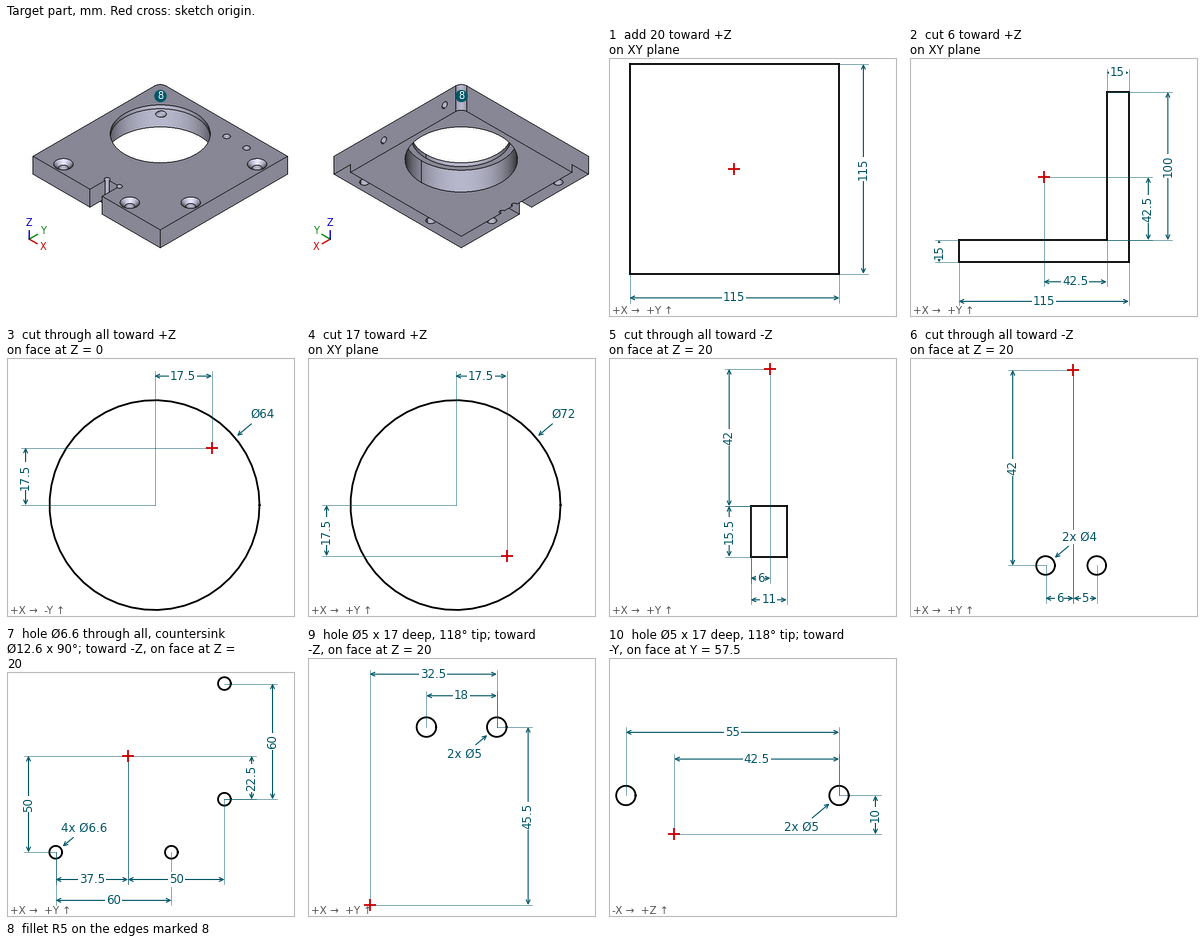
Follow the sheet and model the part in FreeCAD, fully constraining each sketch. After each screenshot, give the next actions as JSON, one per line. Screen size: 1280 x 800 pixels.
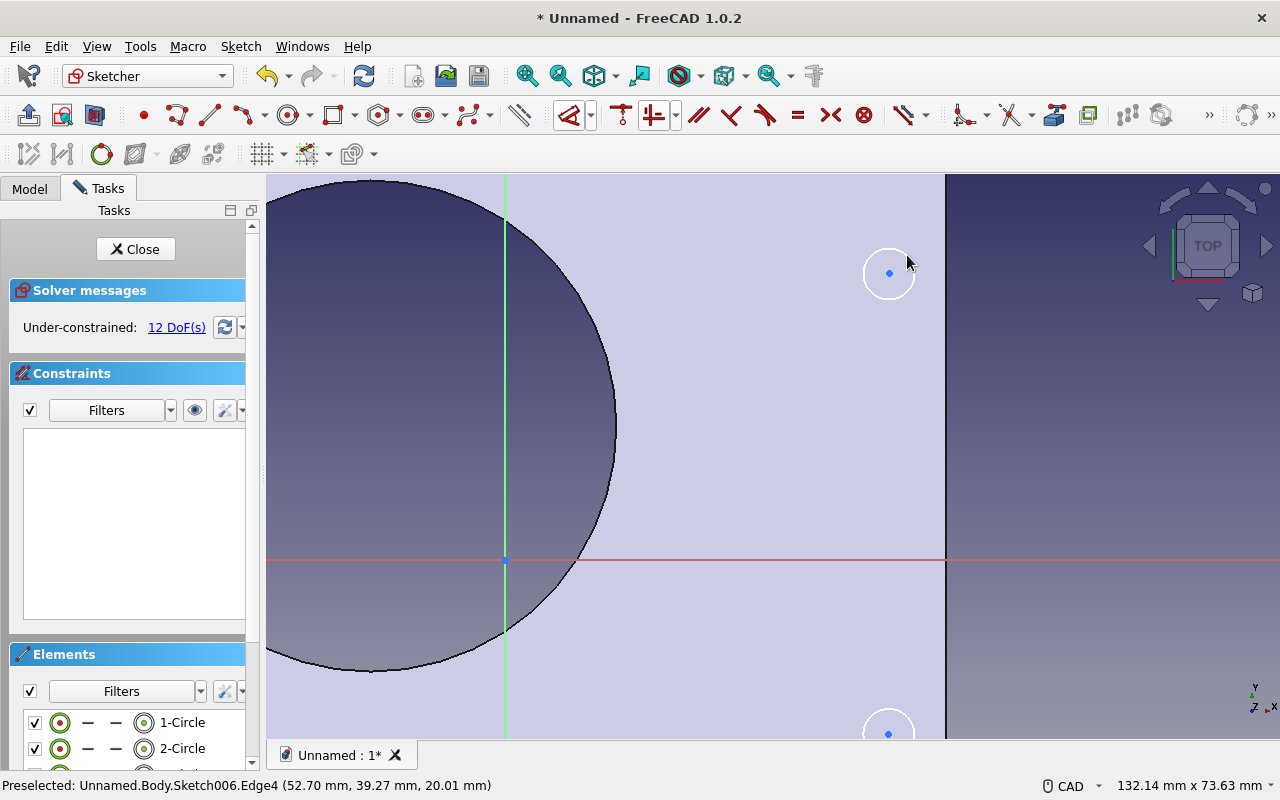
{"action": "scroll", "coordinate": [889, 272], "scroll_direction": "down", "scroll_amount": 3}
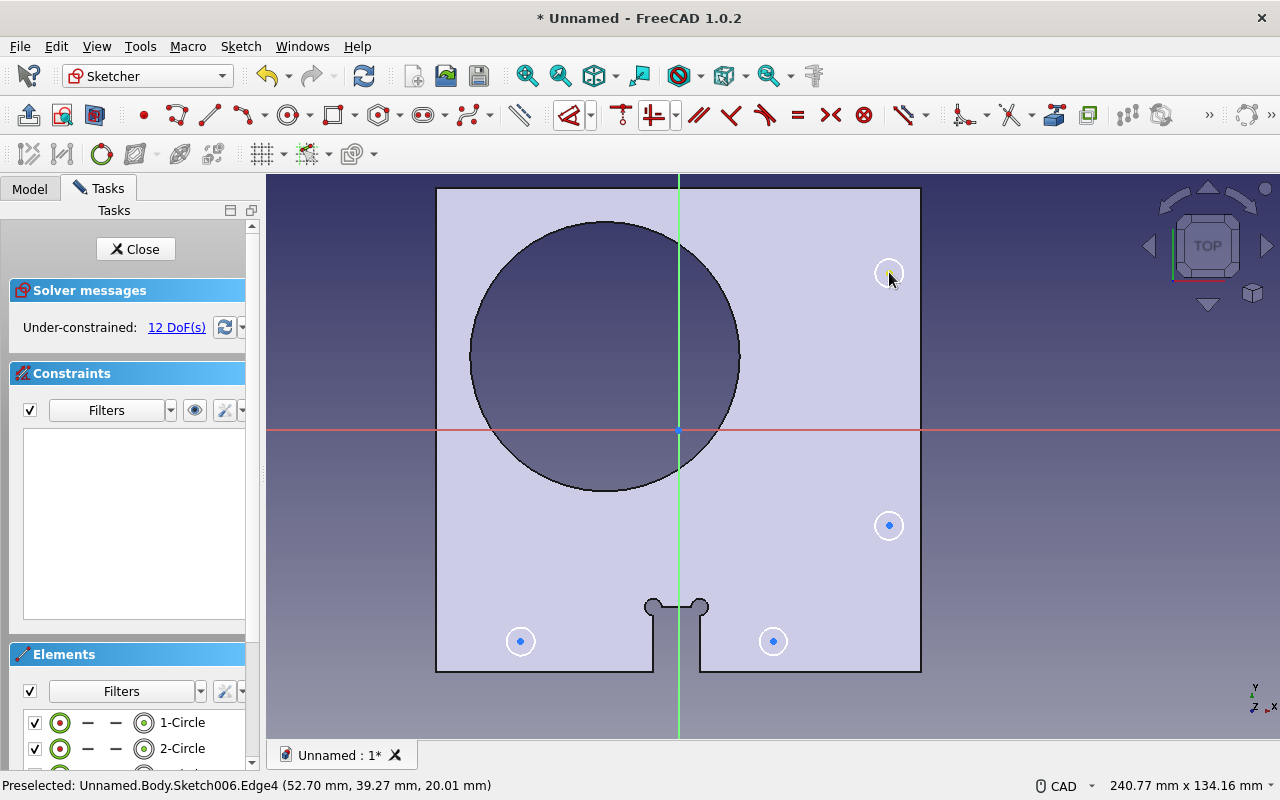
{"action": "left_click", "coordinate": [531, 632]}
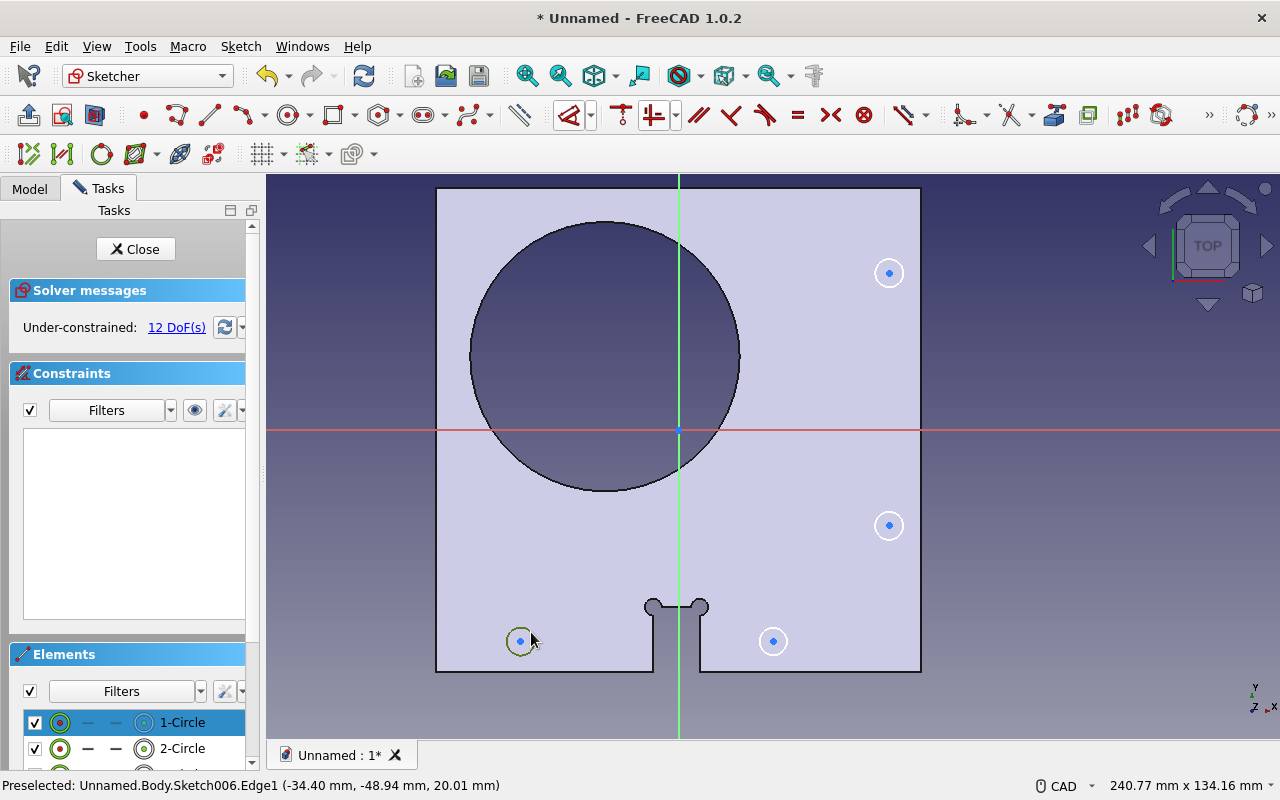
{"action": "left_click", "coordinate": [783, 632]}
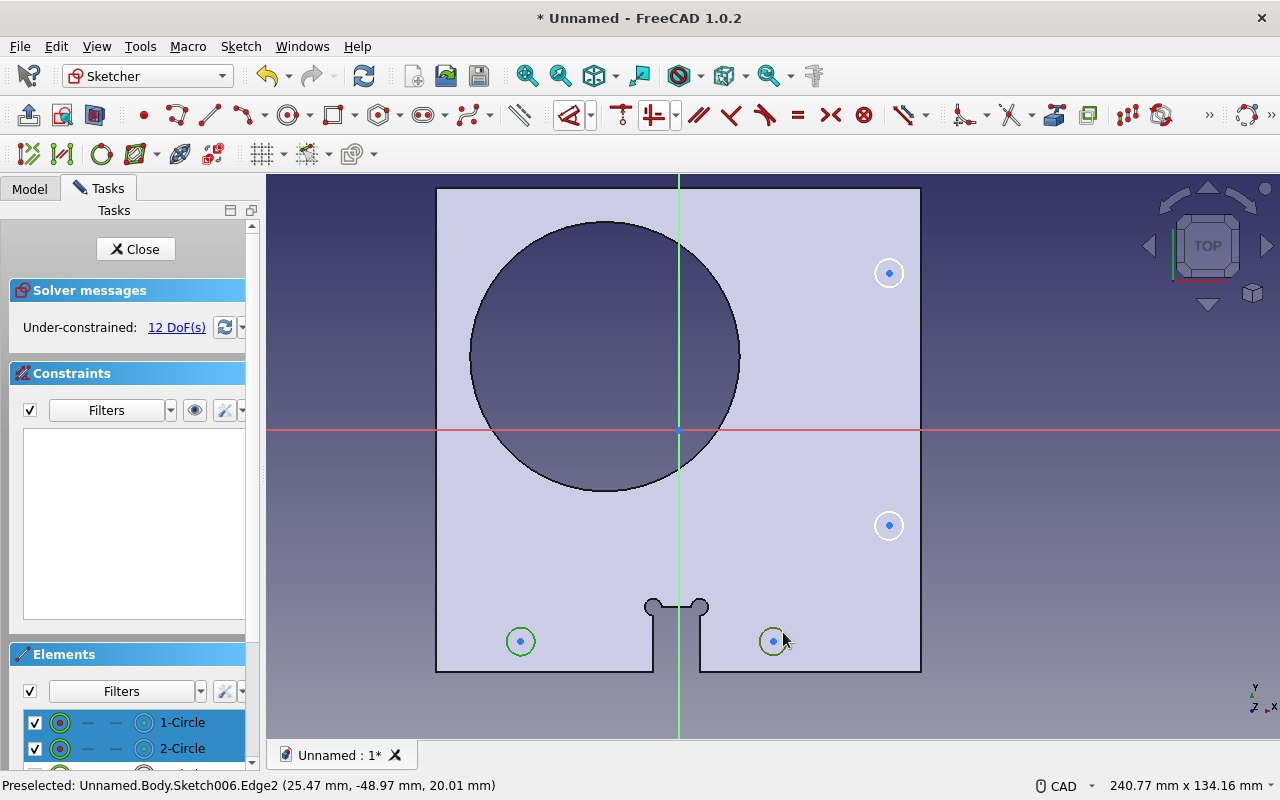
{"action": "left_click", "coordinate": [899, 516]}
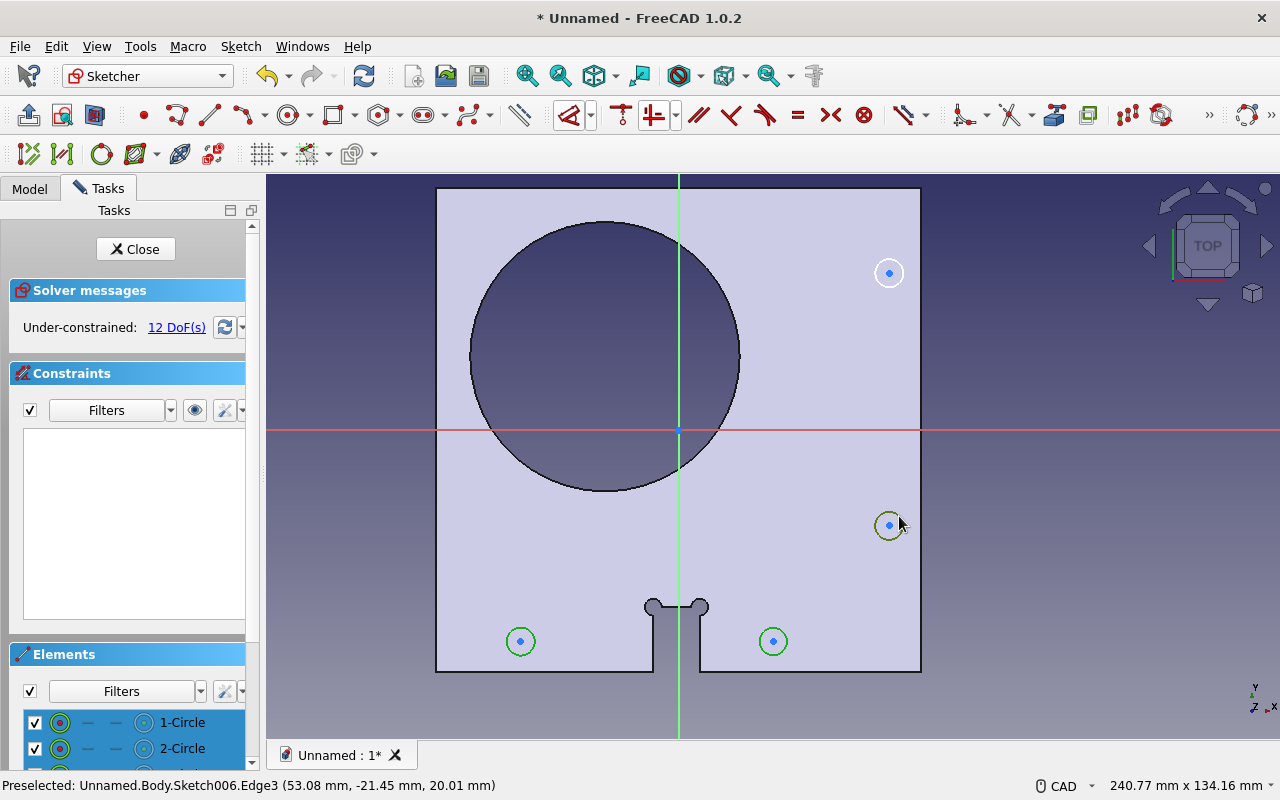
{"action": "left_click", "coordinate": [899, 263]}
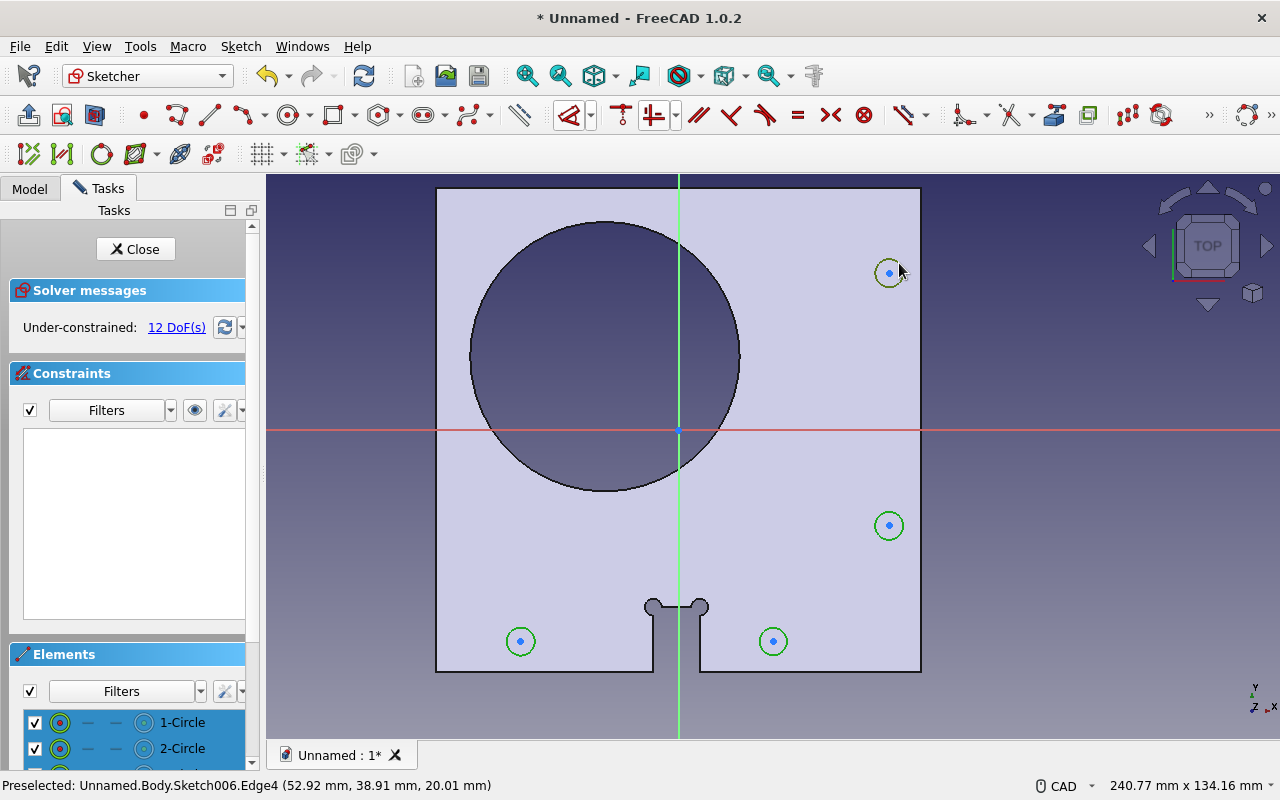
{"action": "key", "text": "e"}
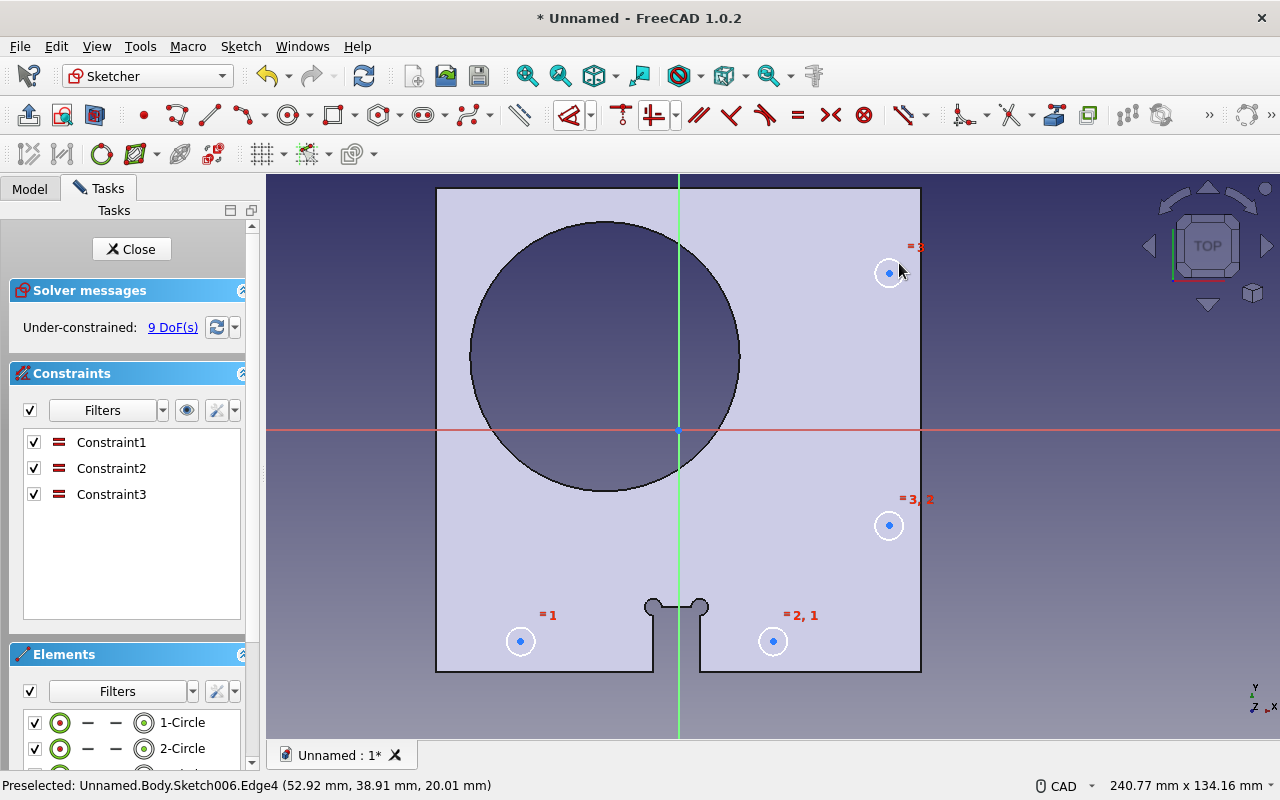
{"action": "left_click", "coordinate": [521, 642]}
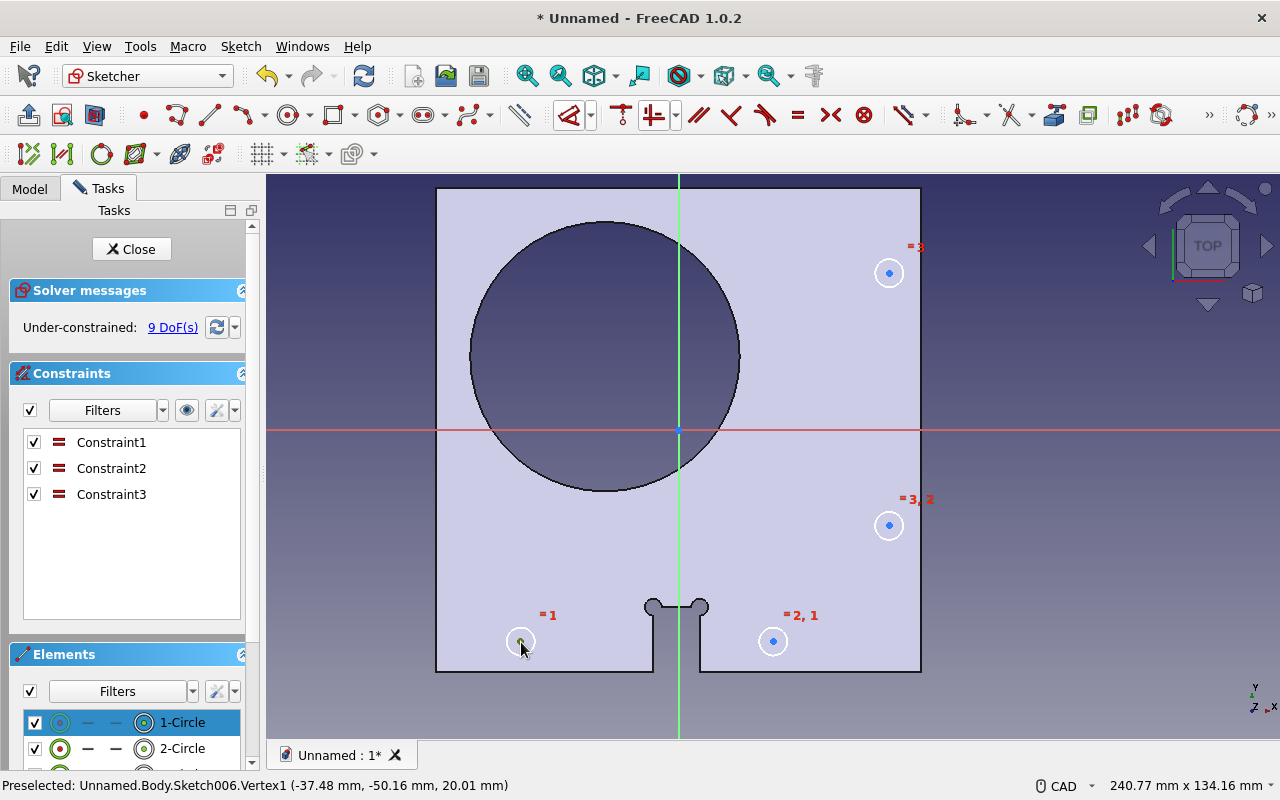
{"action": "left_click", "coordinate": [773, 642]}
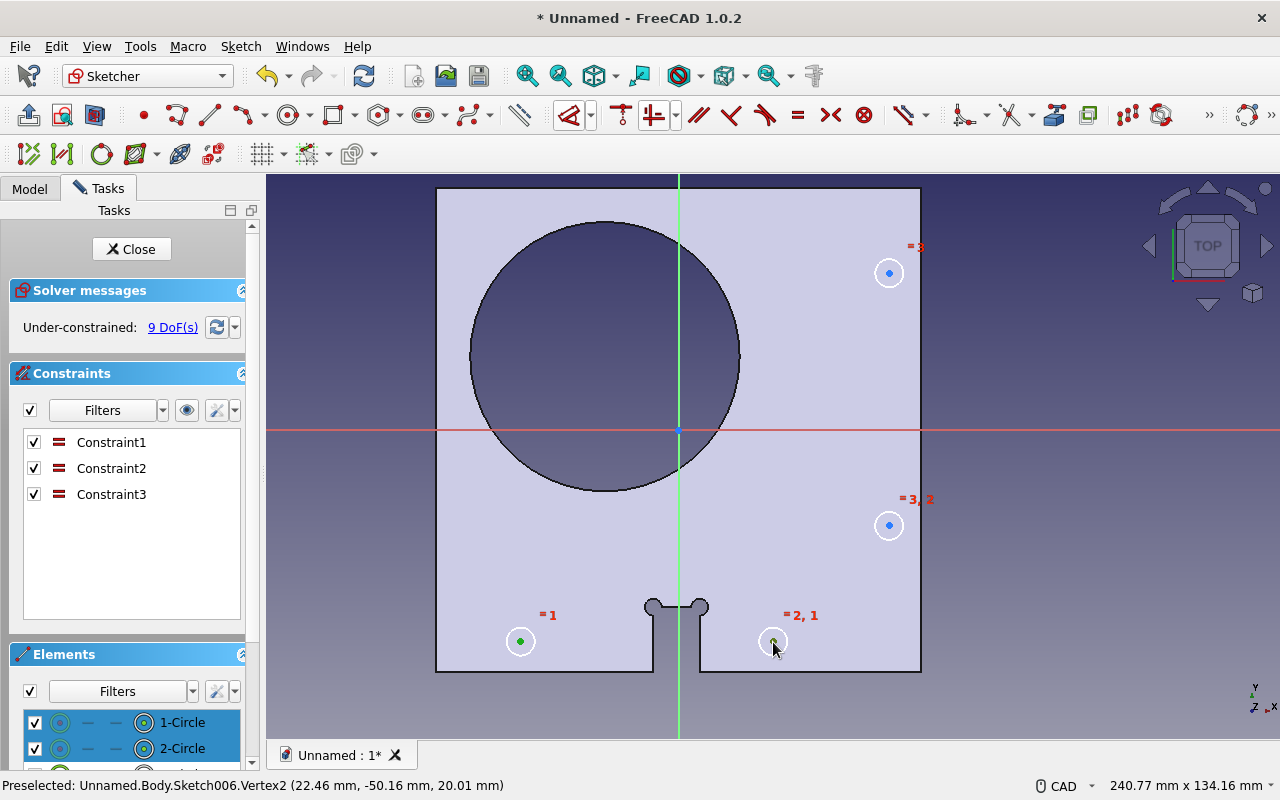
{"action": "key", "text": "h"}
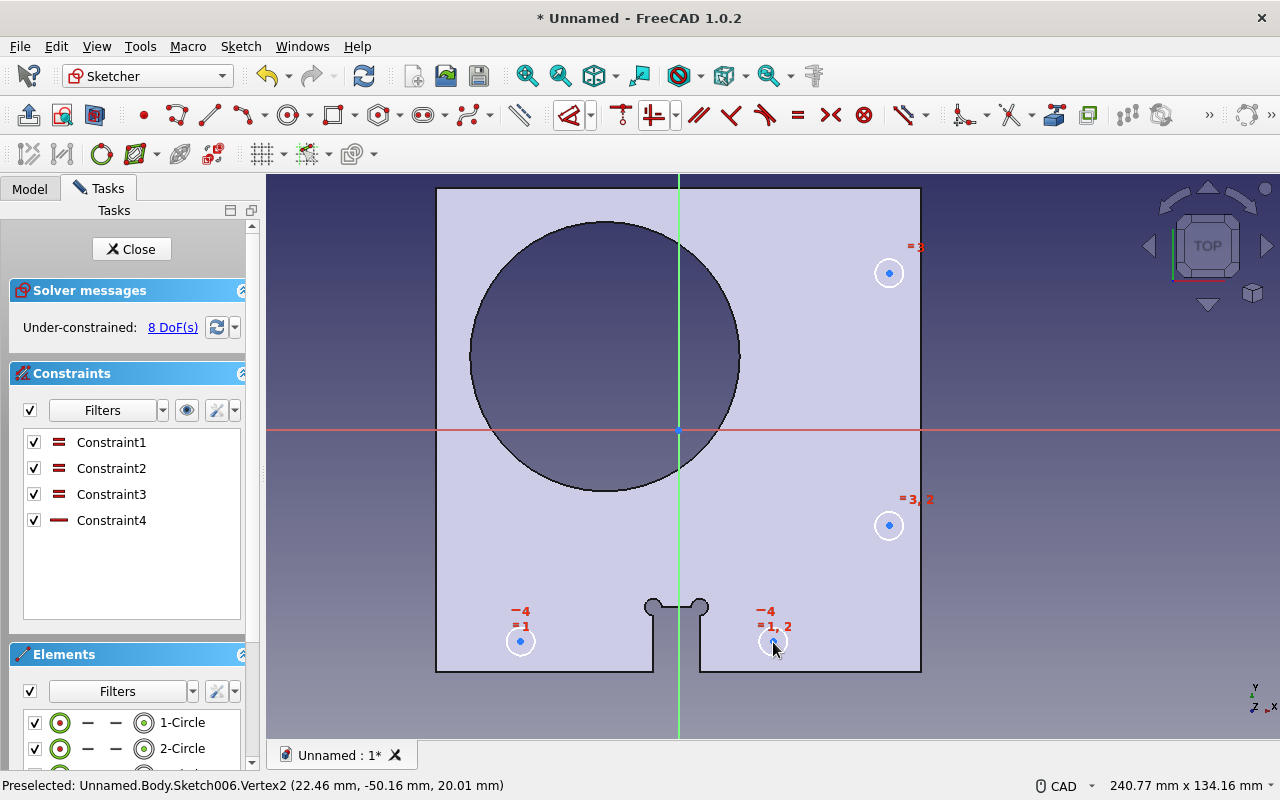
{"action": "left_click", "coordinate": [889, 526]}